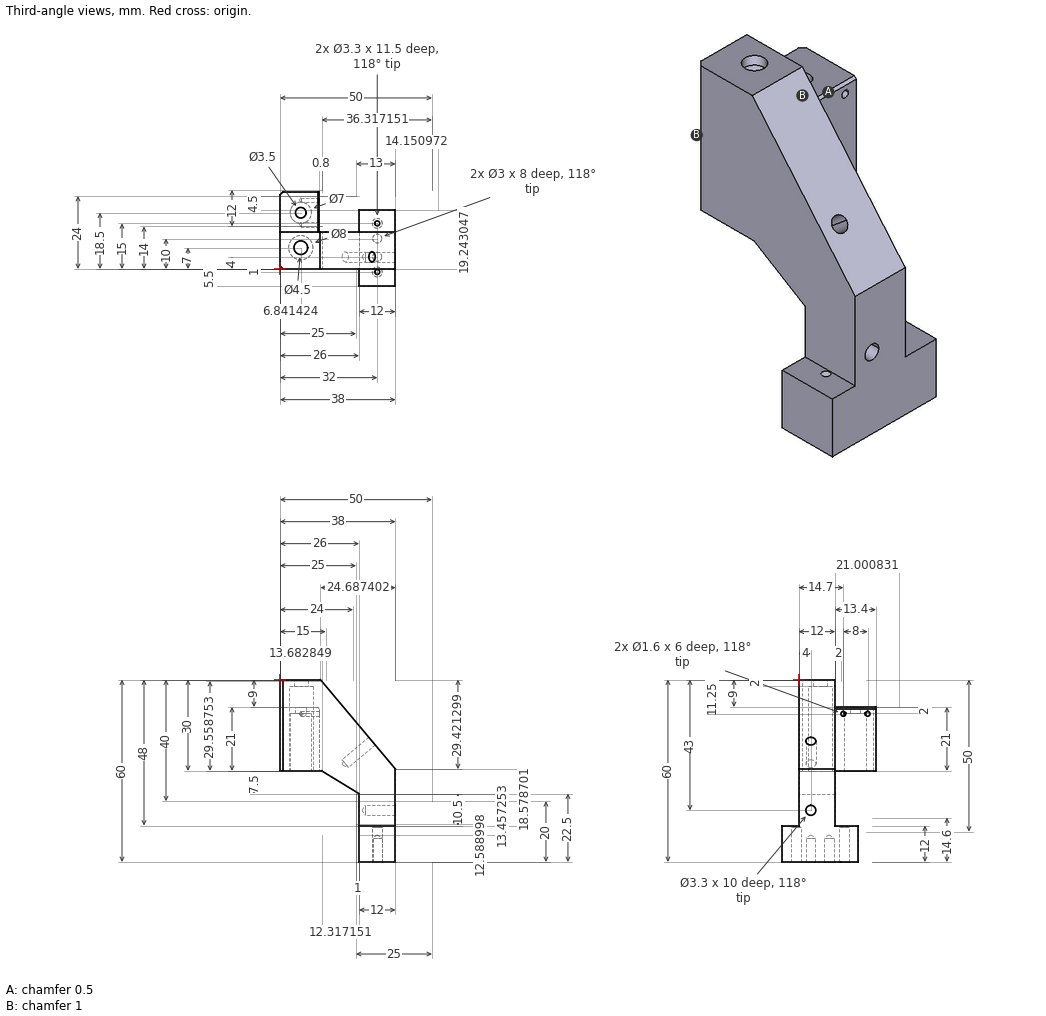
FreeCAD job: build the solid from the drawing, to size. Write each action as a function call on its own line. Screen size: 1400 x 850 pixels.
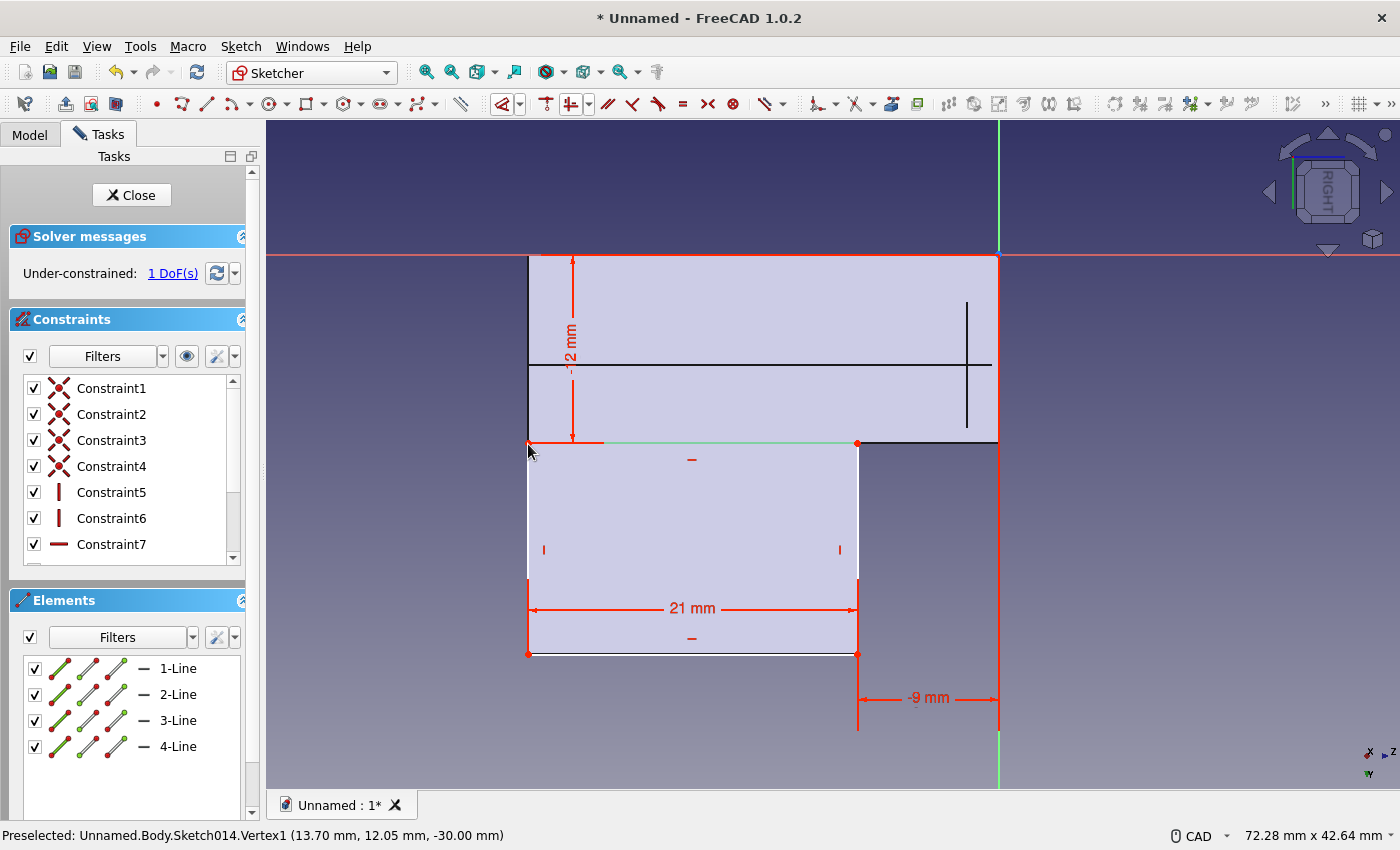
click(528, 507)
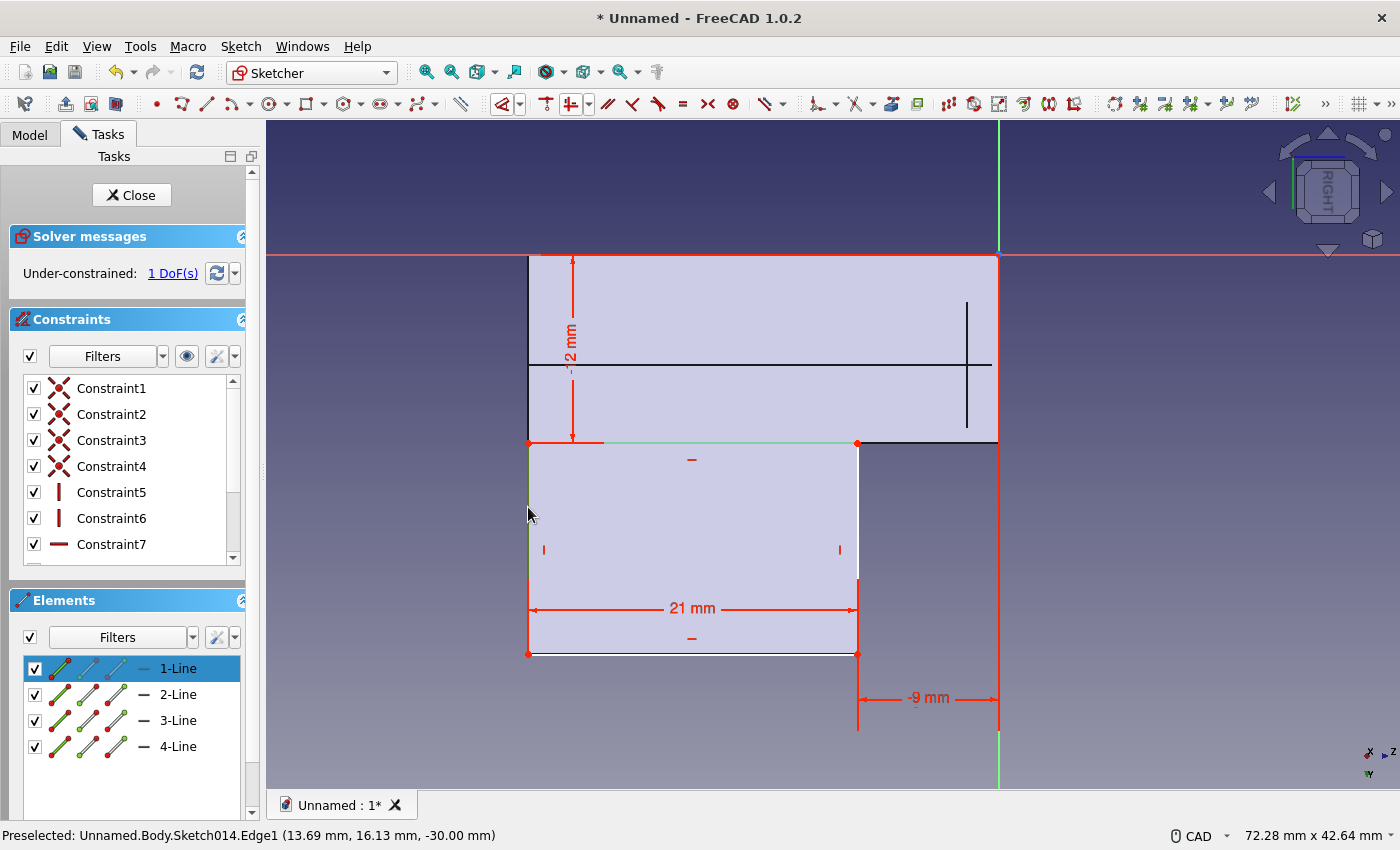
click(520, 104)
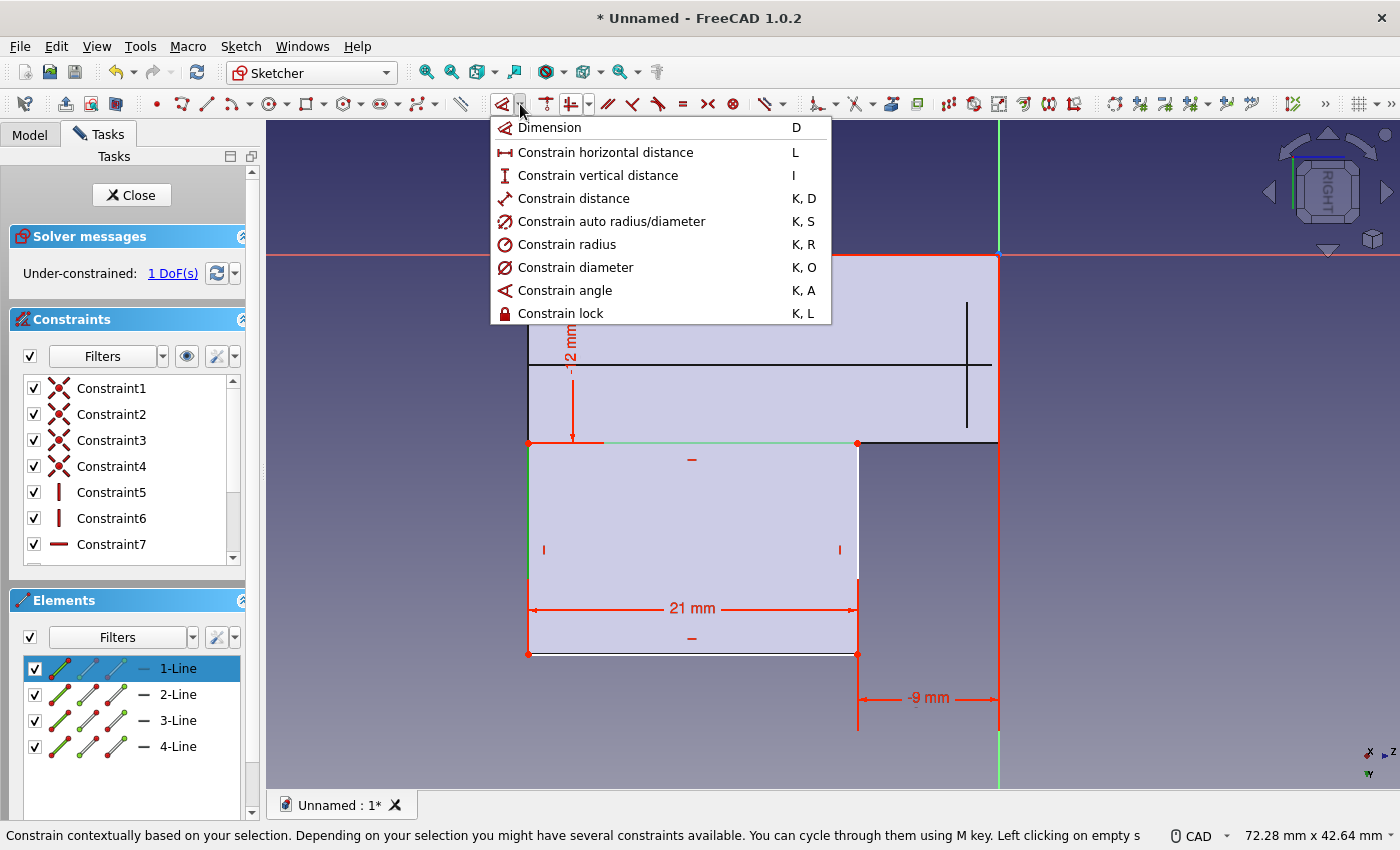
click(661, 176)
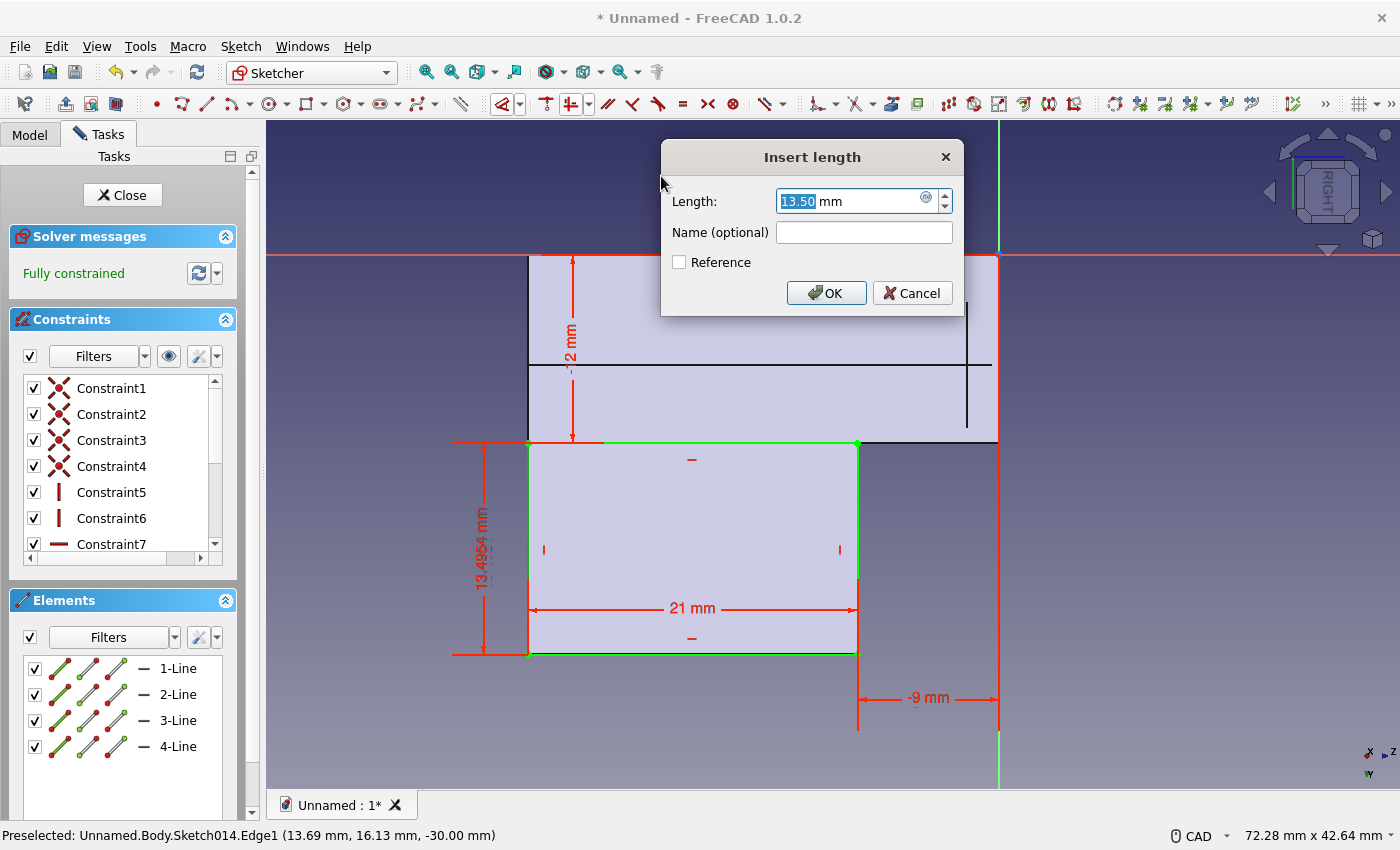
text(13.4)
key(Return)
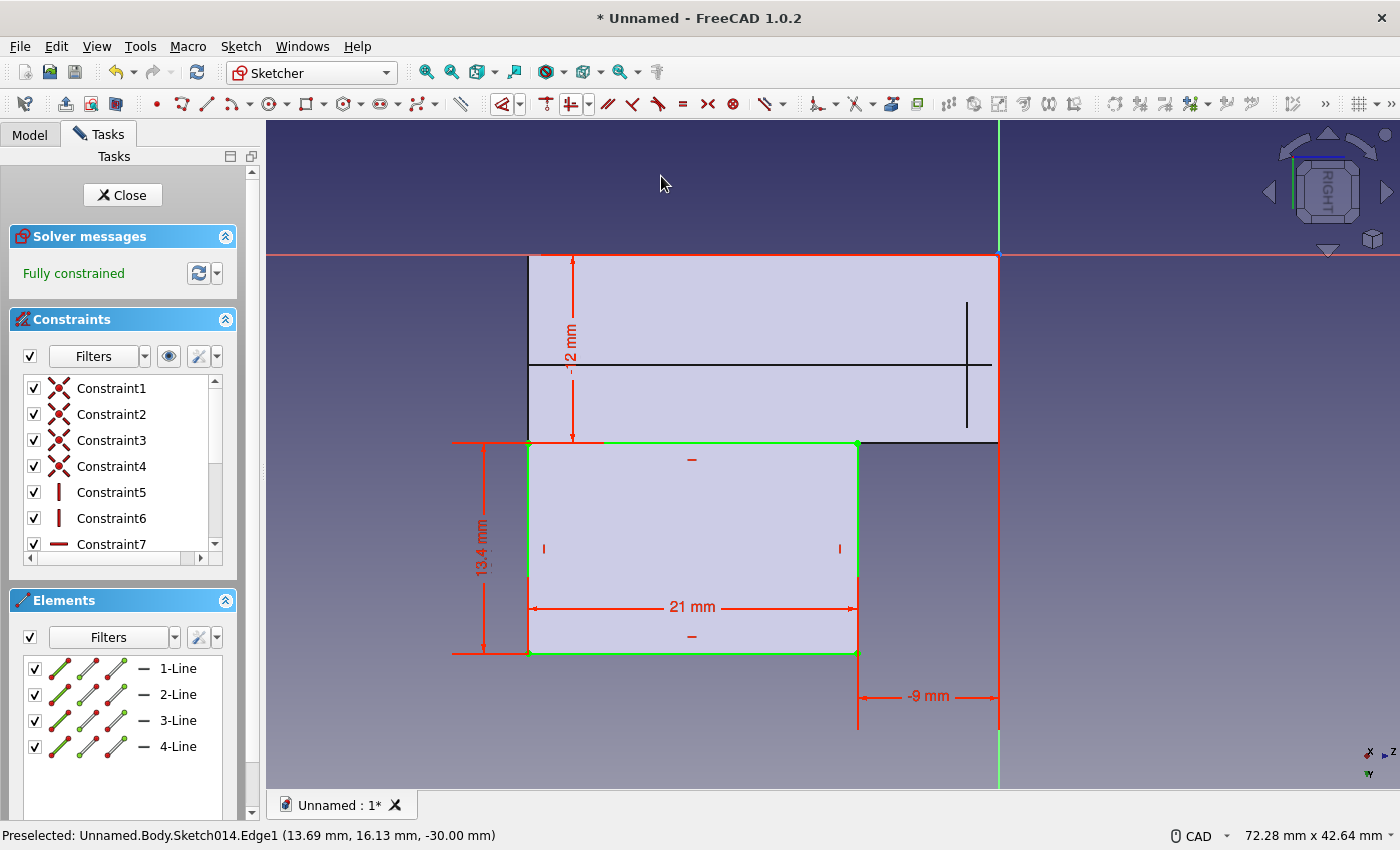
click(123, 195)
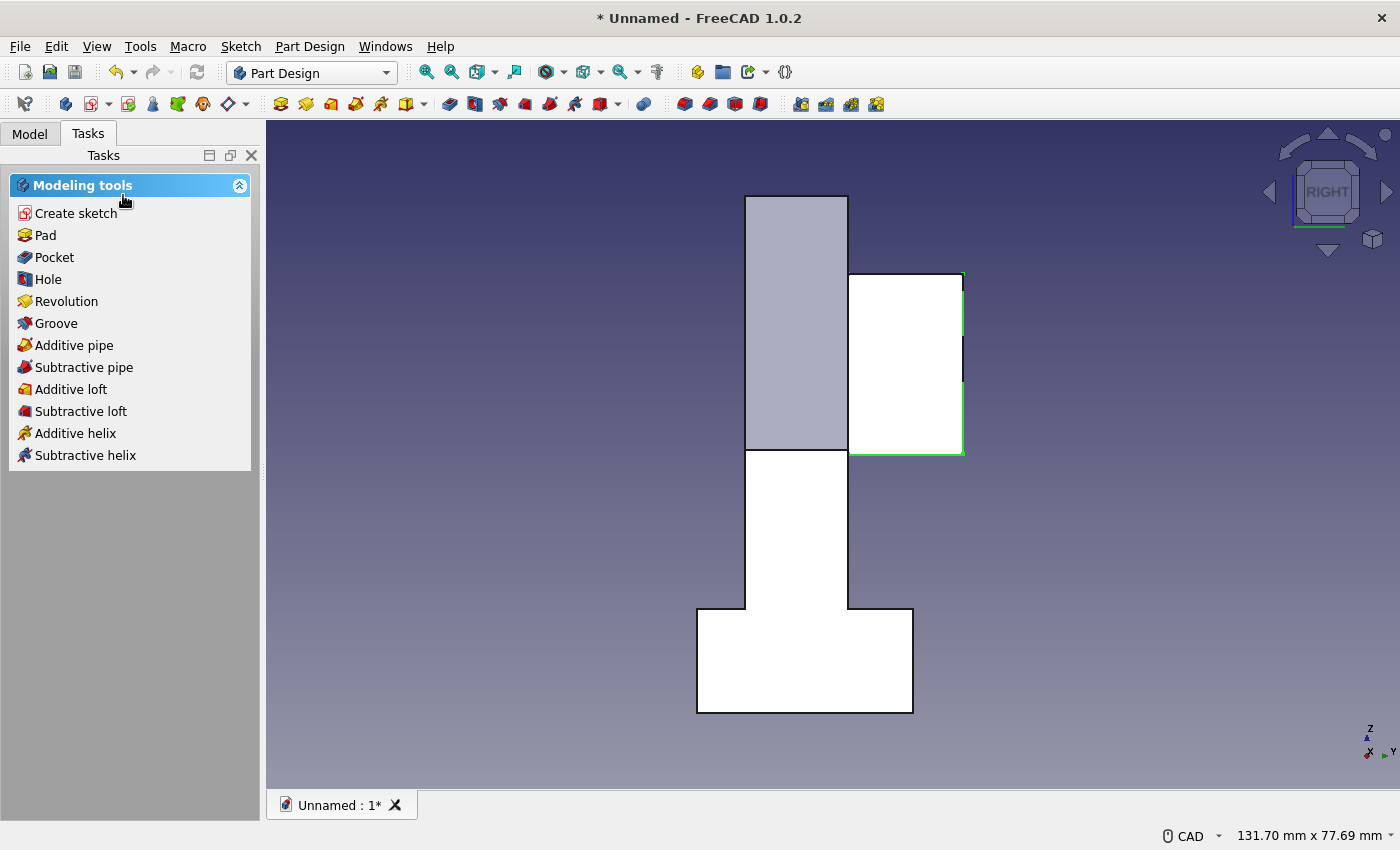
click(450, 104)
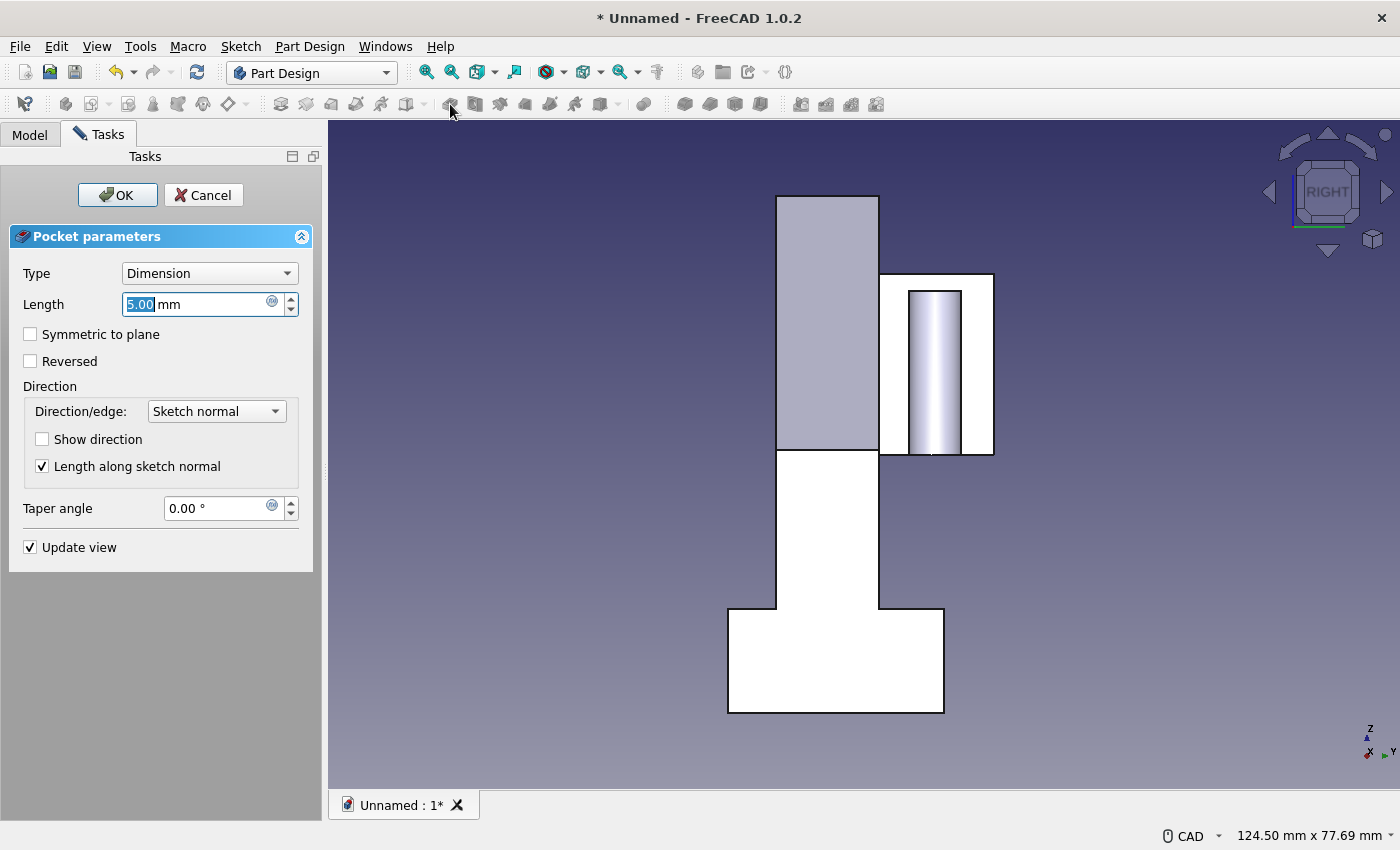
text(0.8)
key(Tab)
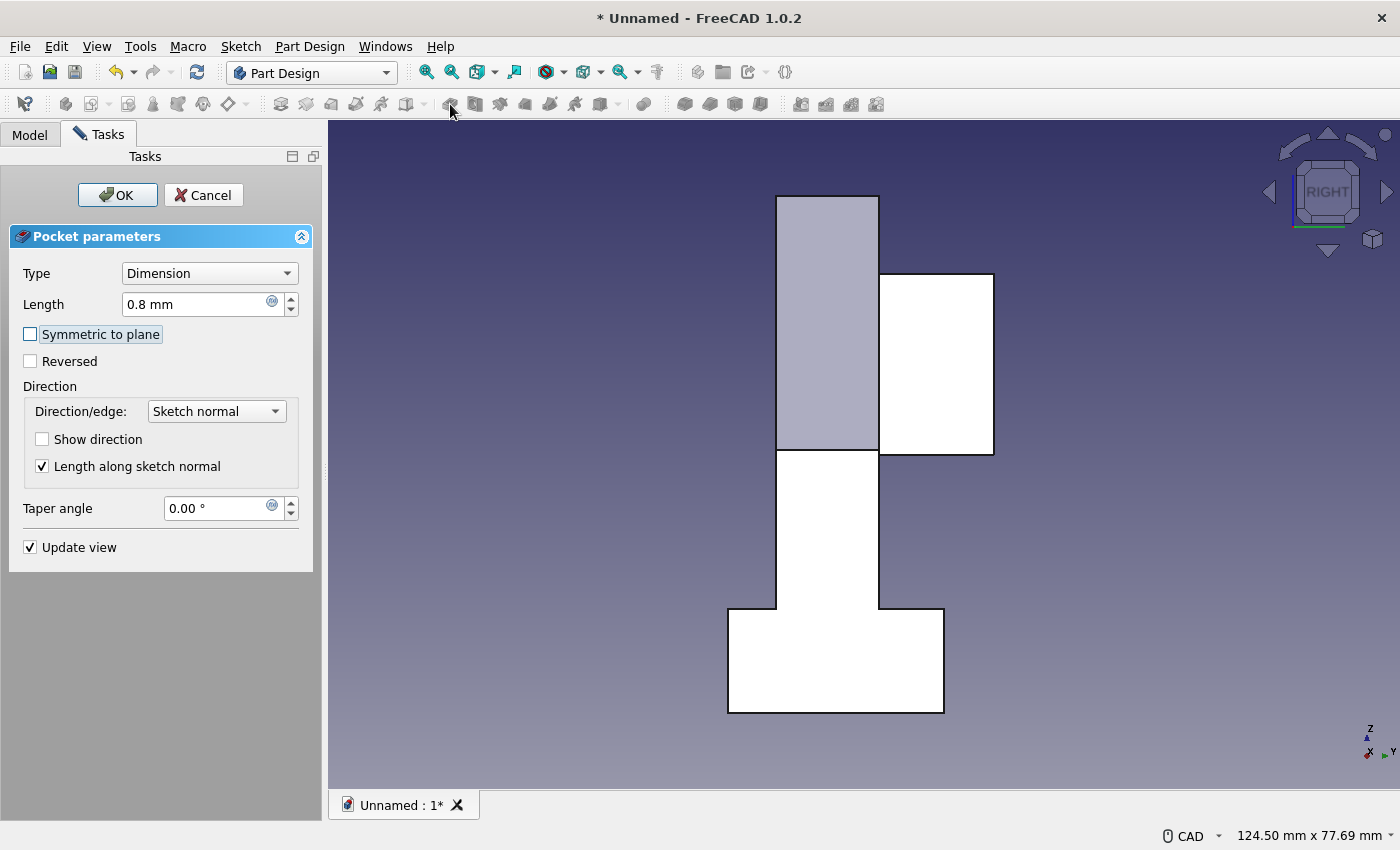
click(118, 195)